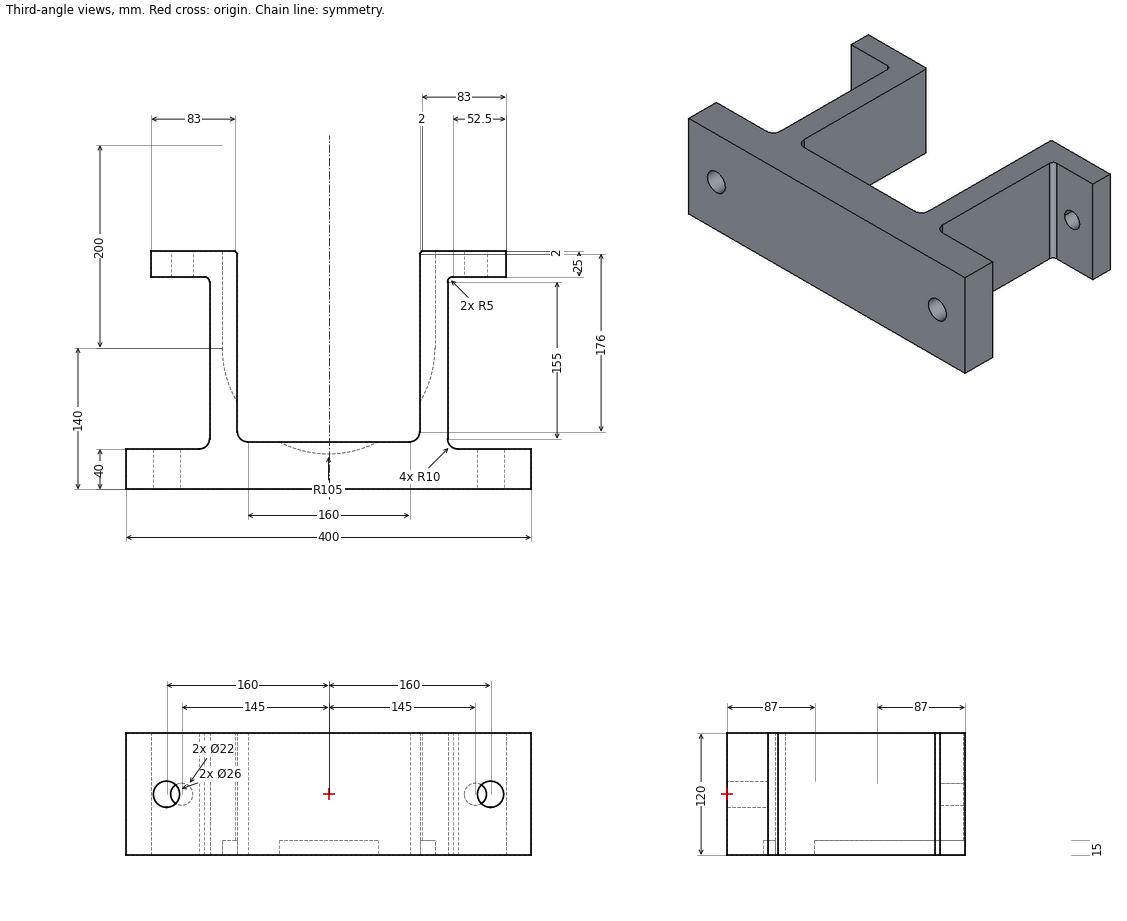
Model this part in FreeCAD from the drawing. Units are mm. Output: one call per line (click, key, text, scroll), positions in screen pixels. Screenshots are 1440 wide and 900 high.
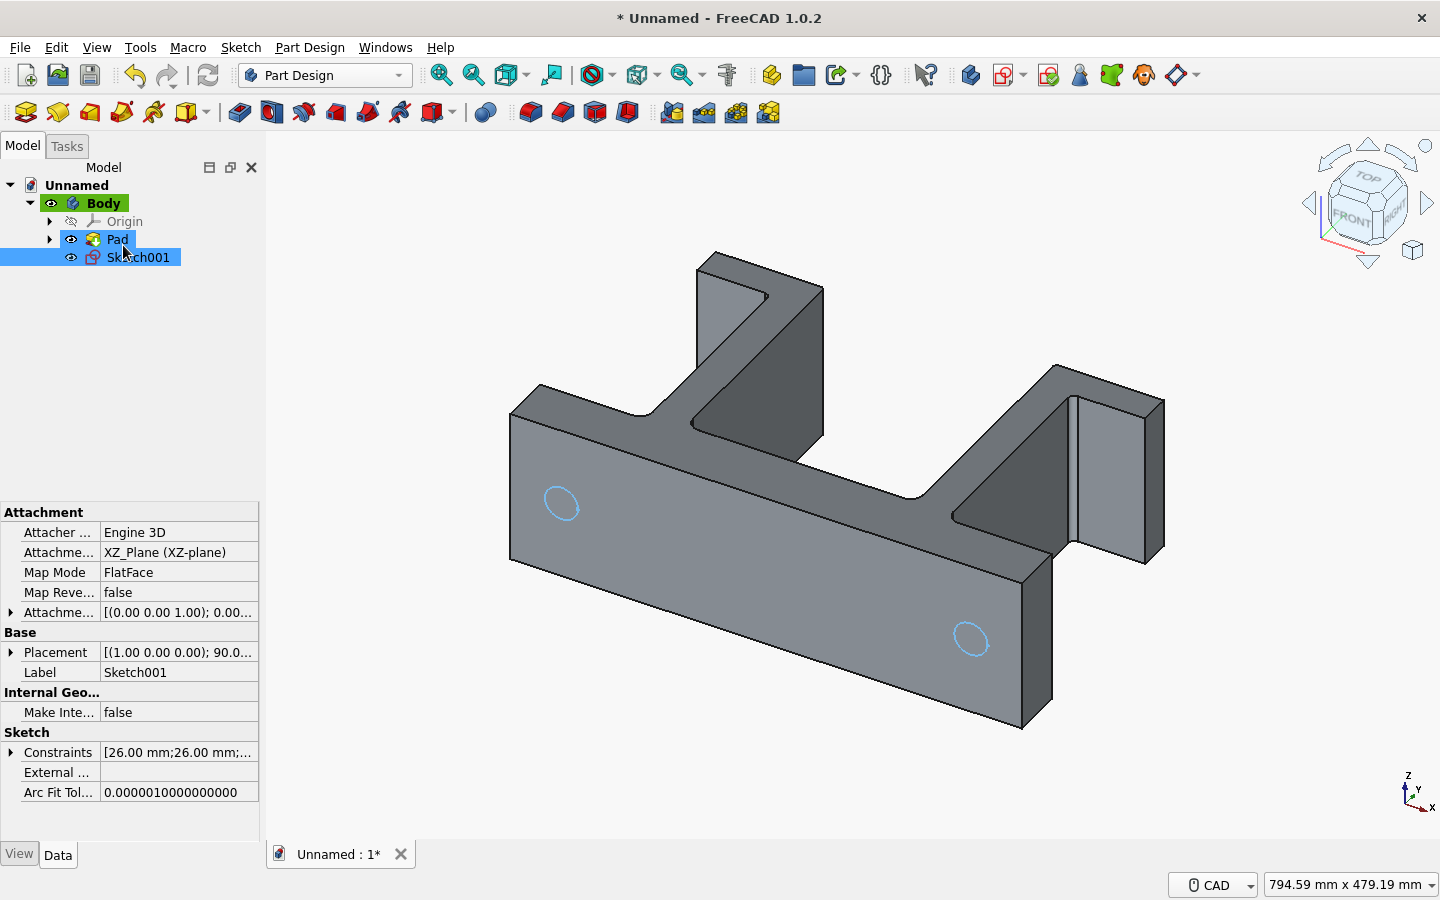
click(240, 112)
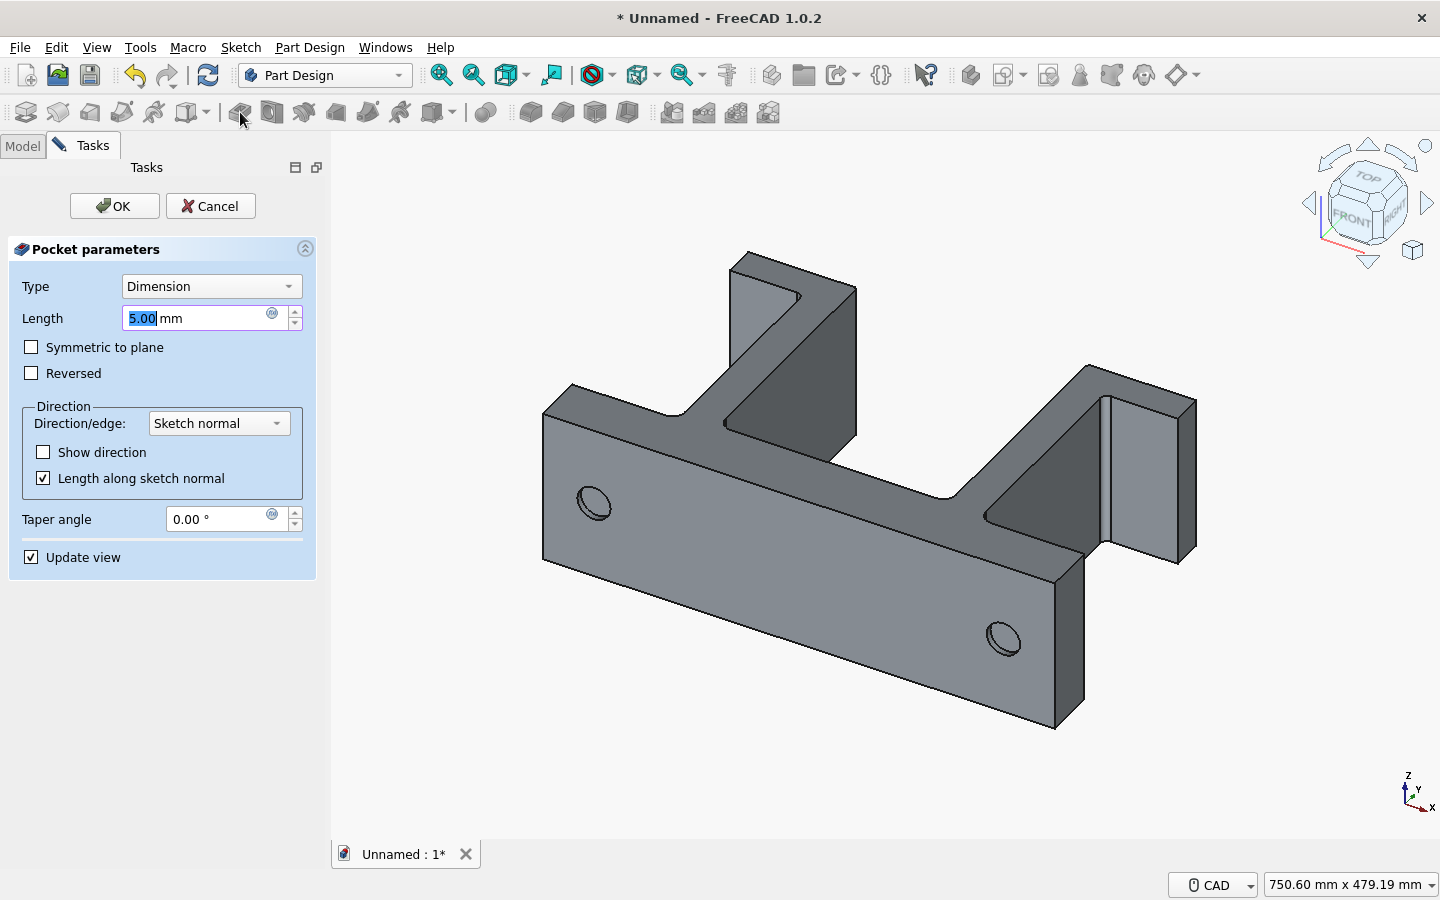
text(87)
key(Tab)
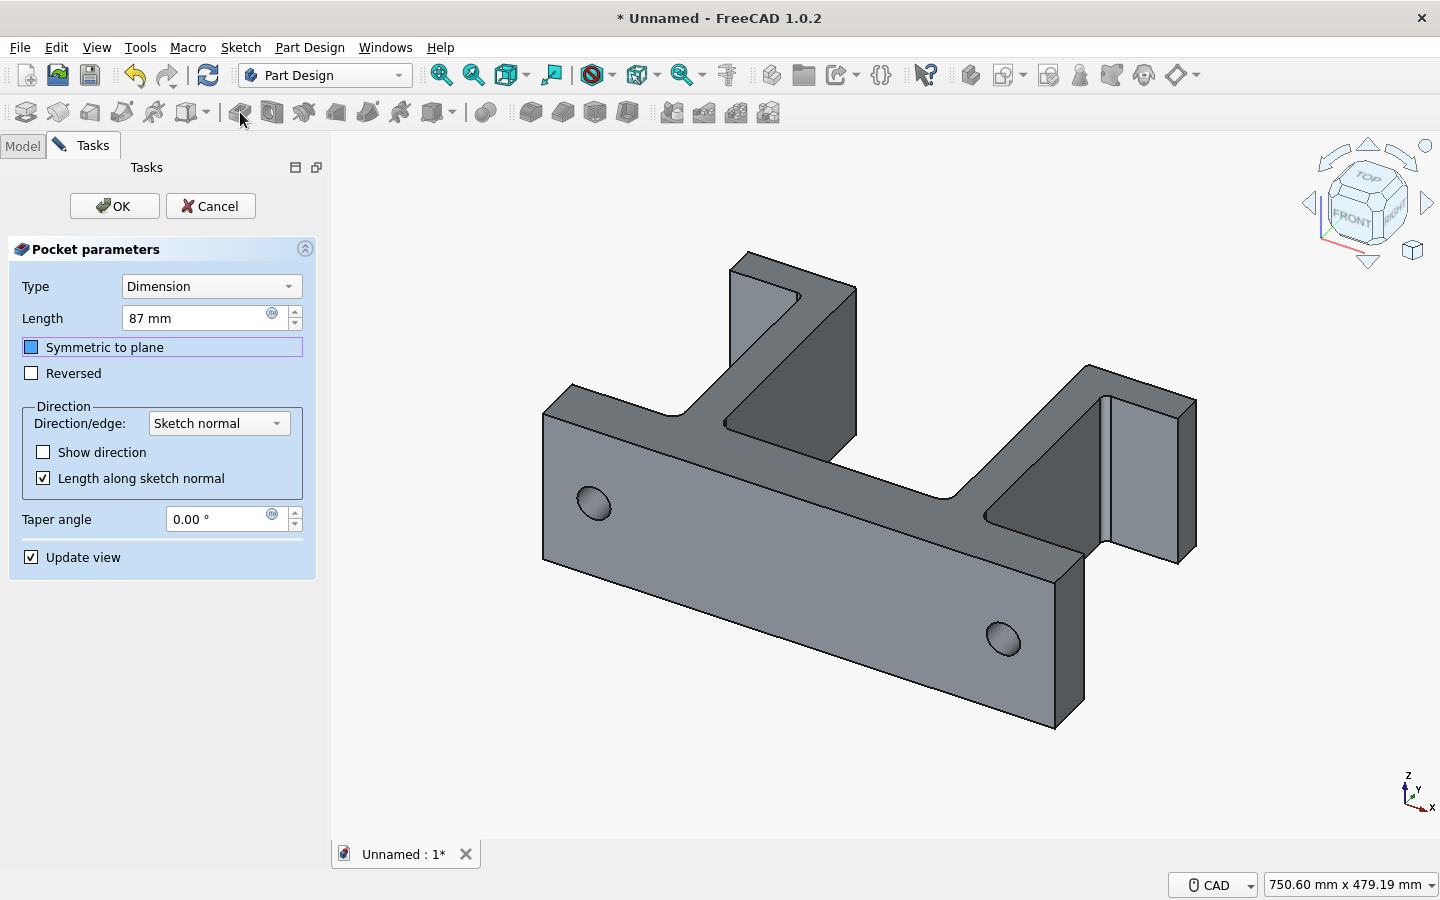
click(115, 206)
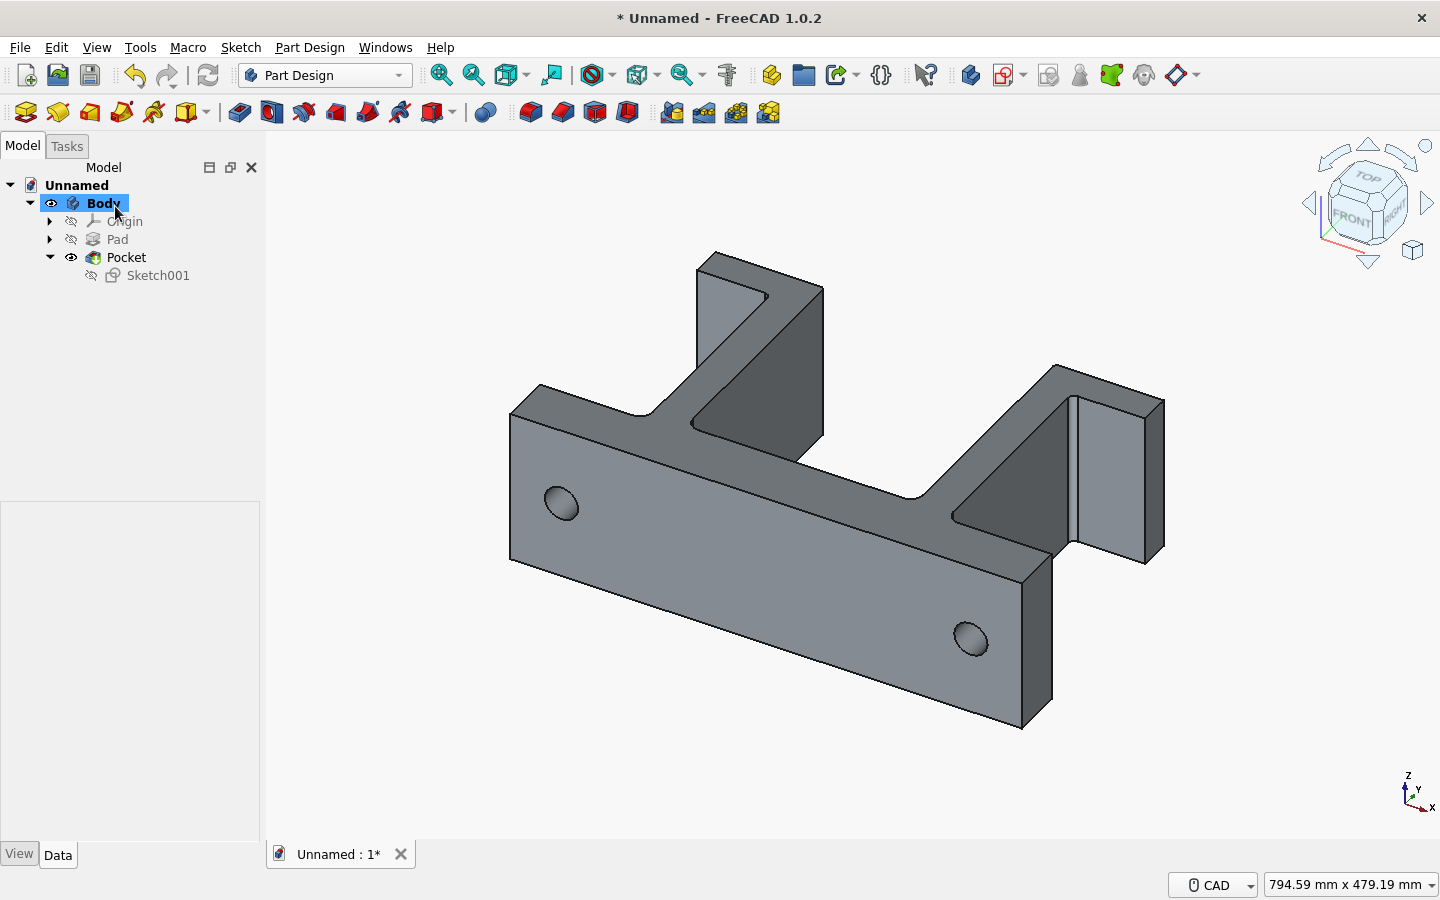
key(4)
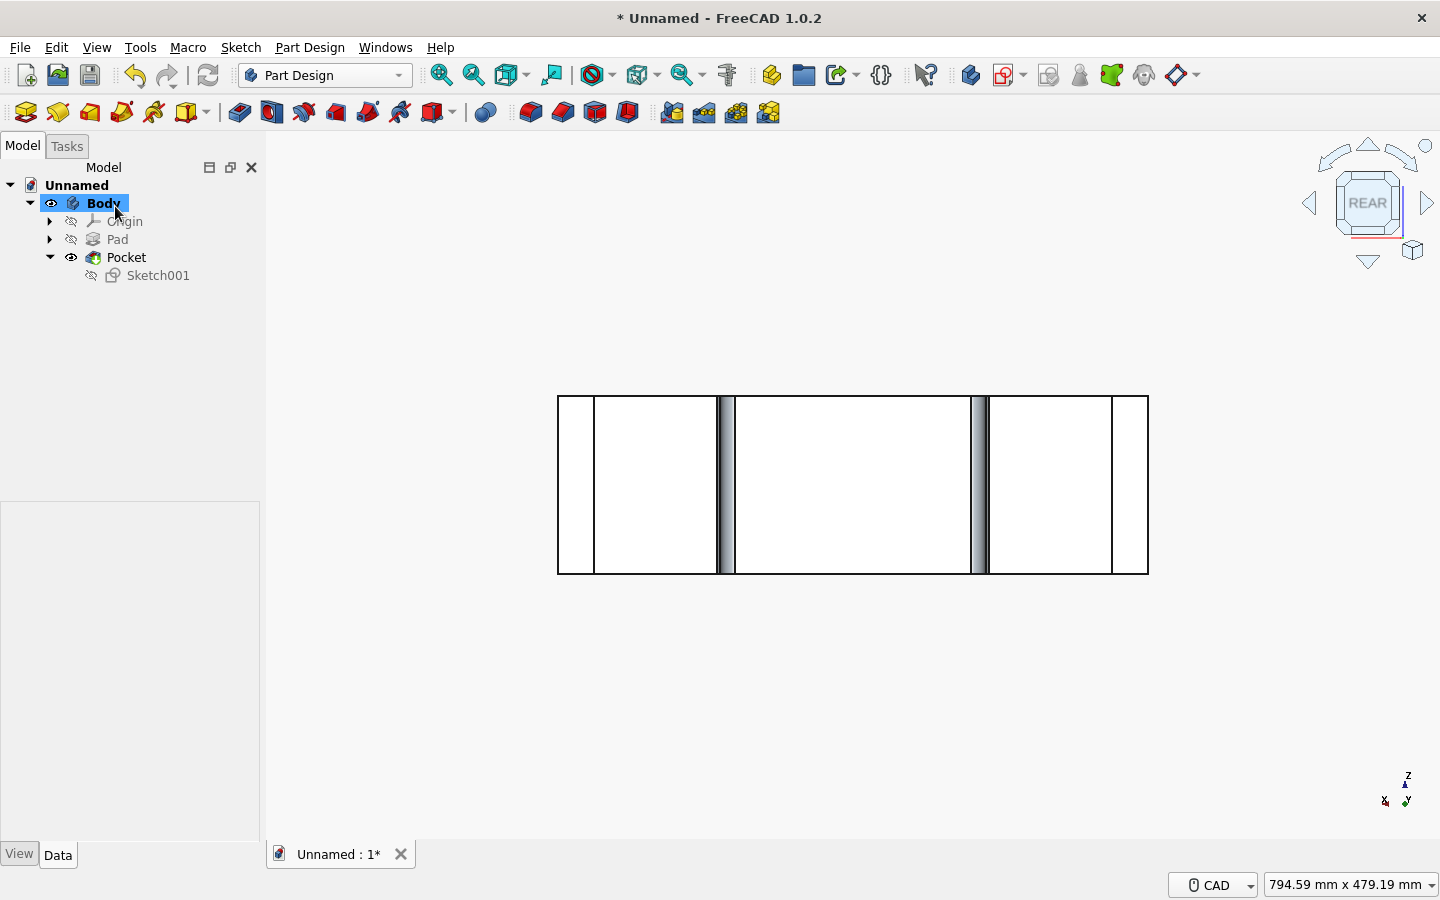
click(656, 459)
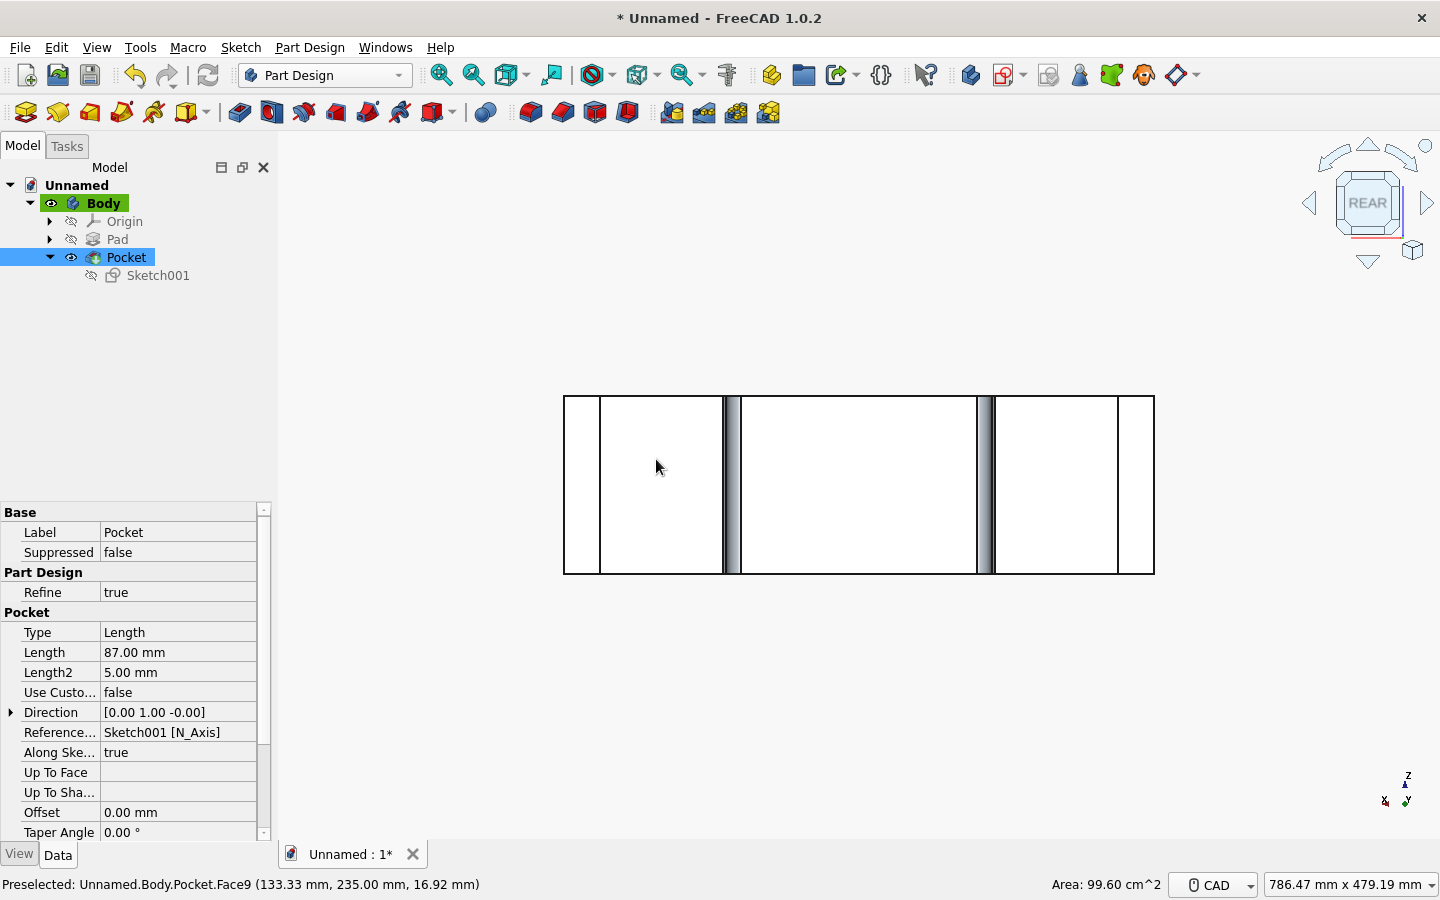
click(1004, 76)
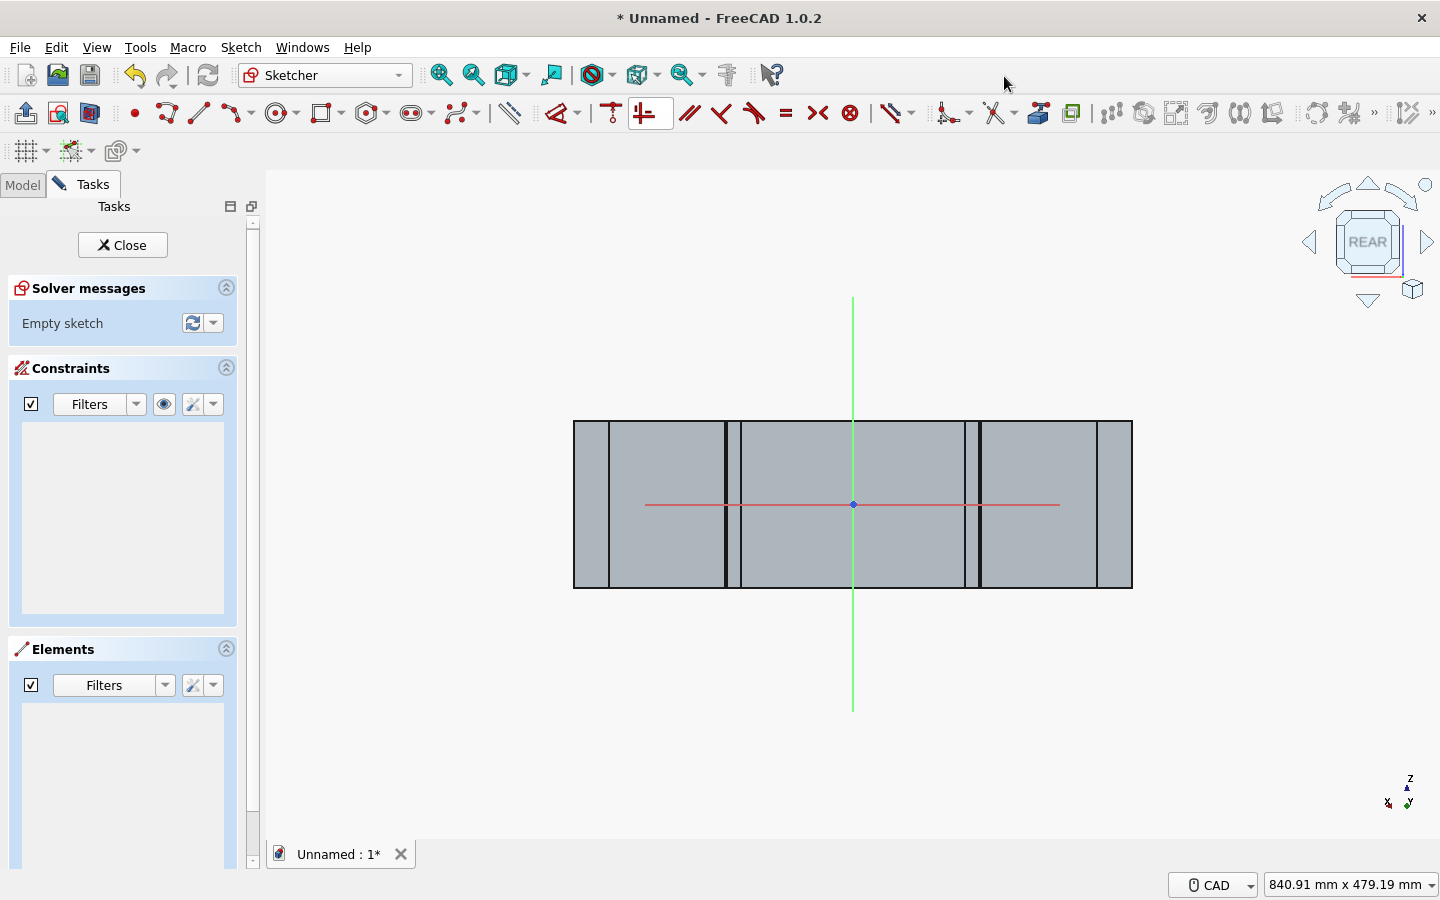
scroll(992, 505, up, 2)